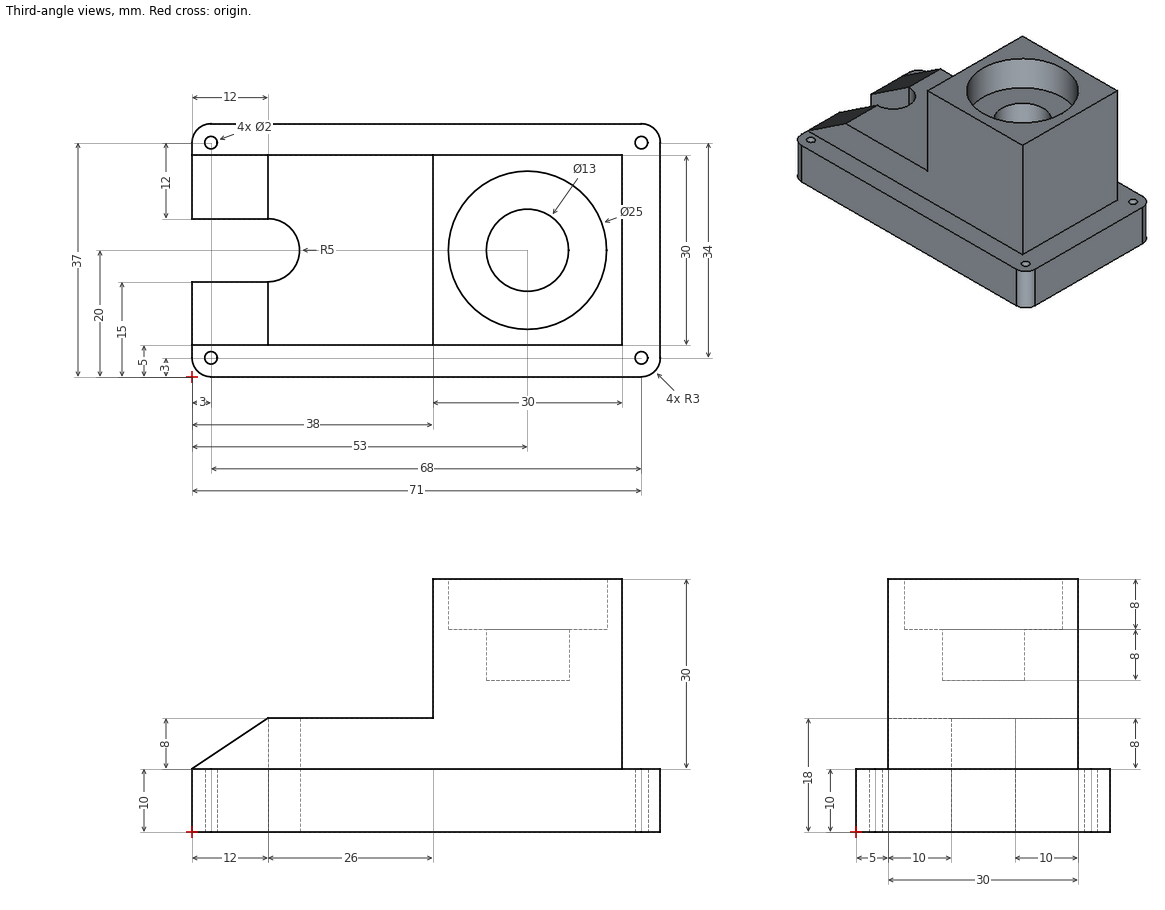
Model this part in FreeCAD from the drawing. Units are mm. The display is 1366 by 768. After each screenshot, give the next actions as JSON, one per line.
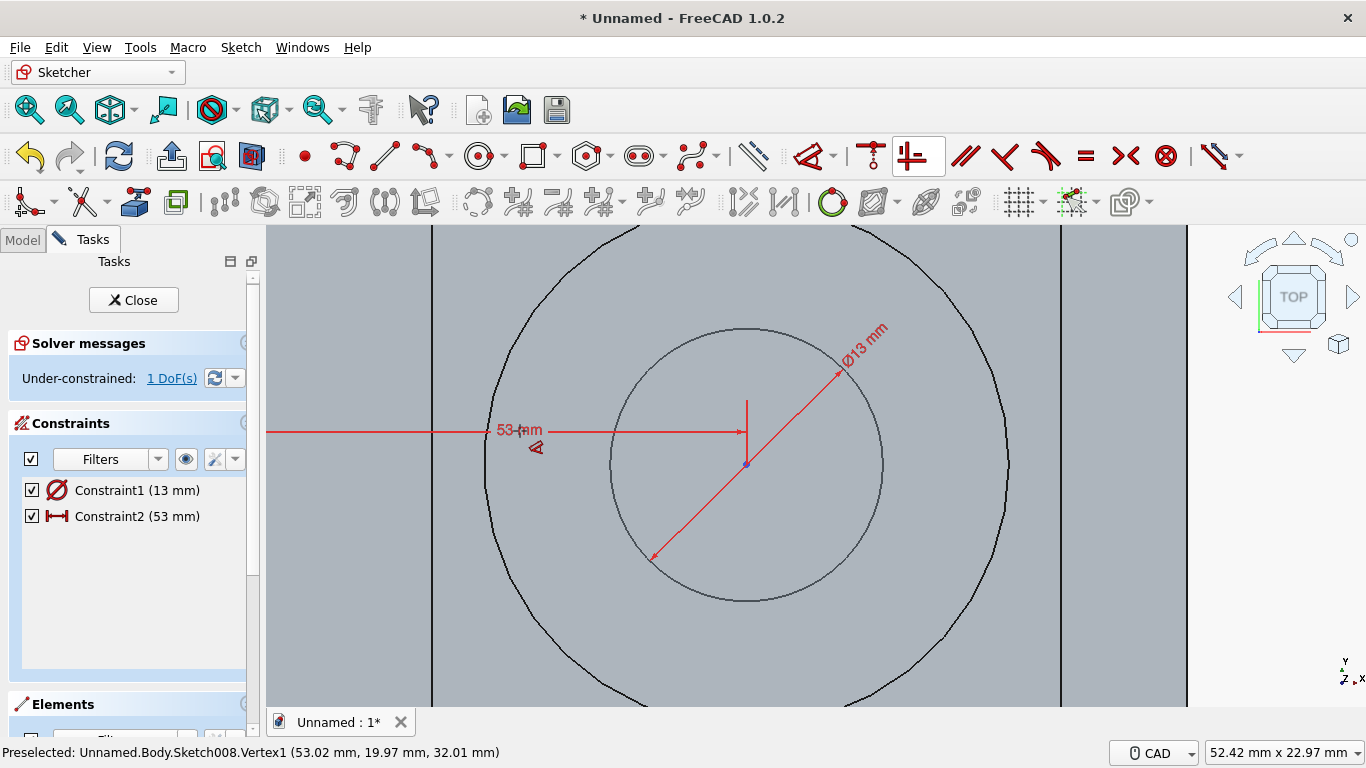
{"action": "left_click", "coordinate": [747, 465]}
{"action": "left_click", "coordinate": [781, 572]}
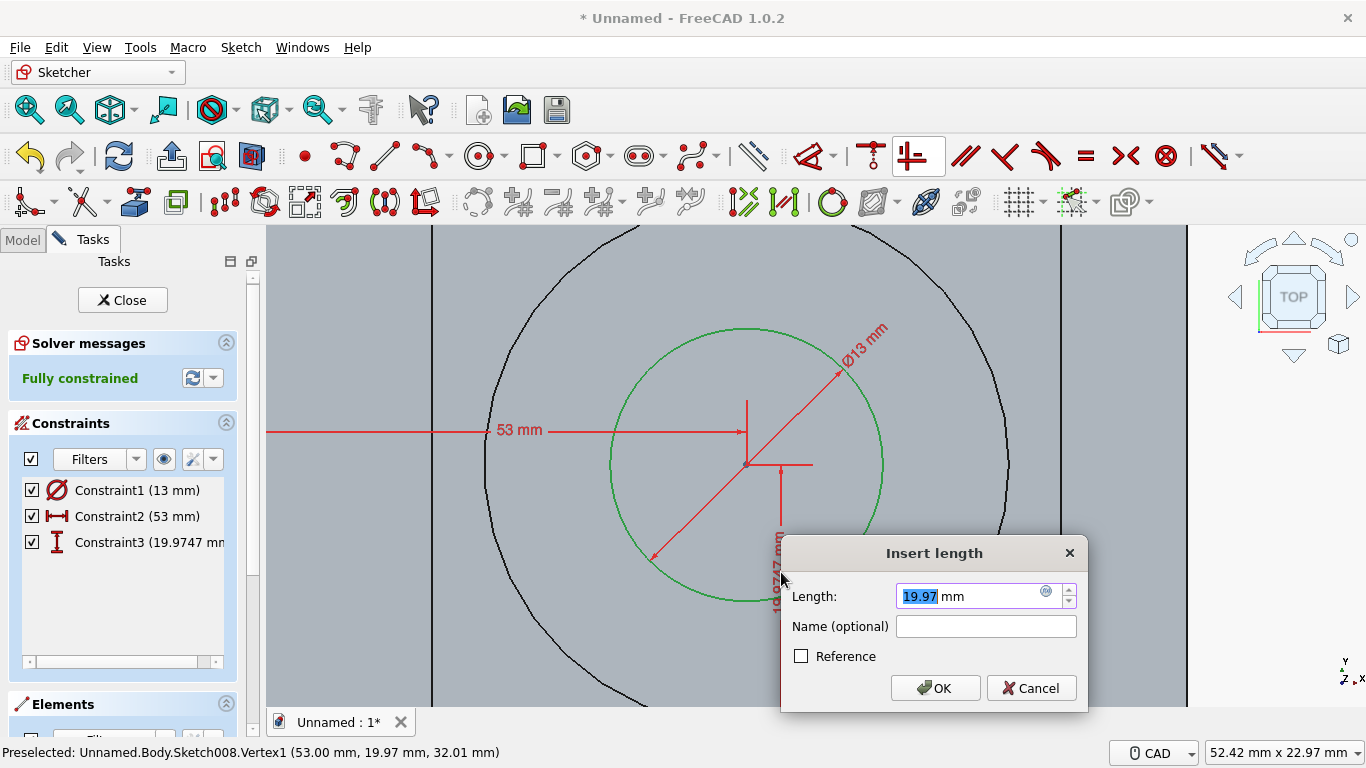
{"action": "type", "text": "20"}
{"action": "key", "text": "Return"}
{"action": "key", "text": "Escape"}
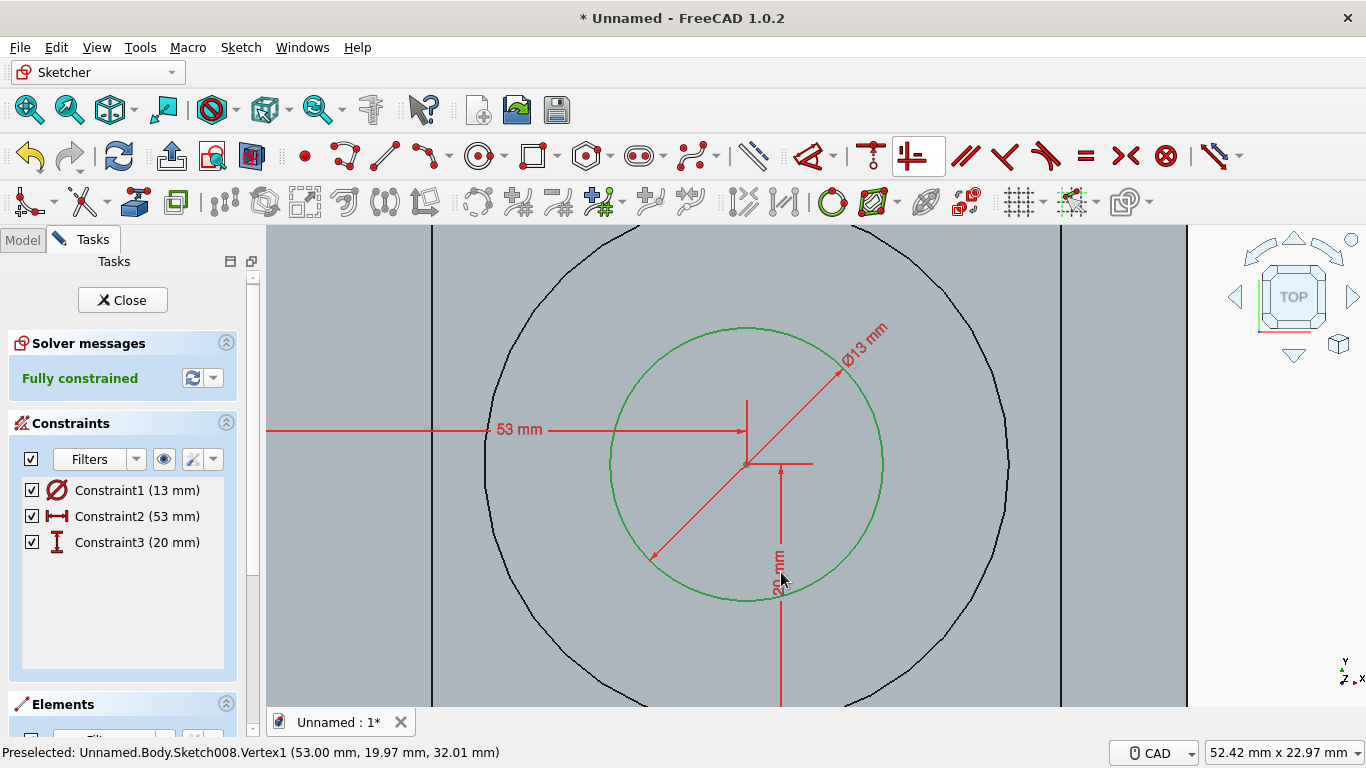
{"action": "left_click", "coordinate": [123, 300]}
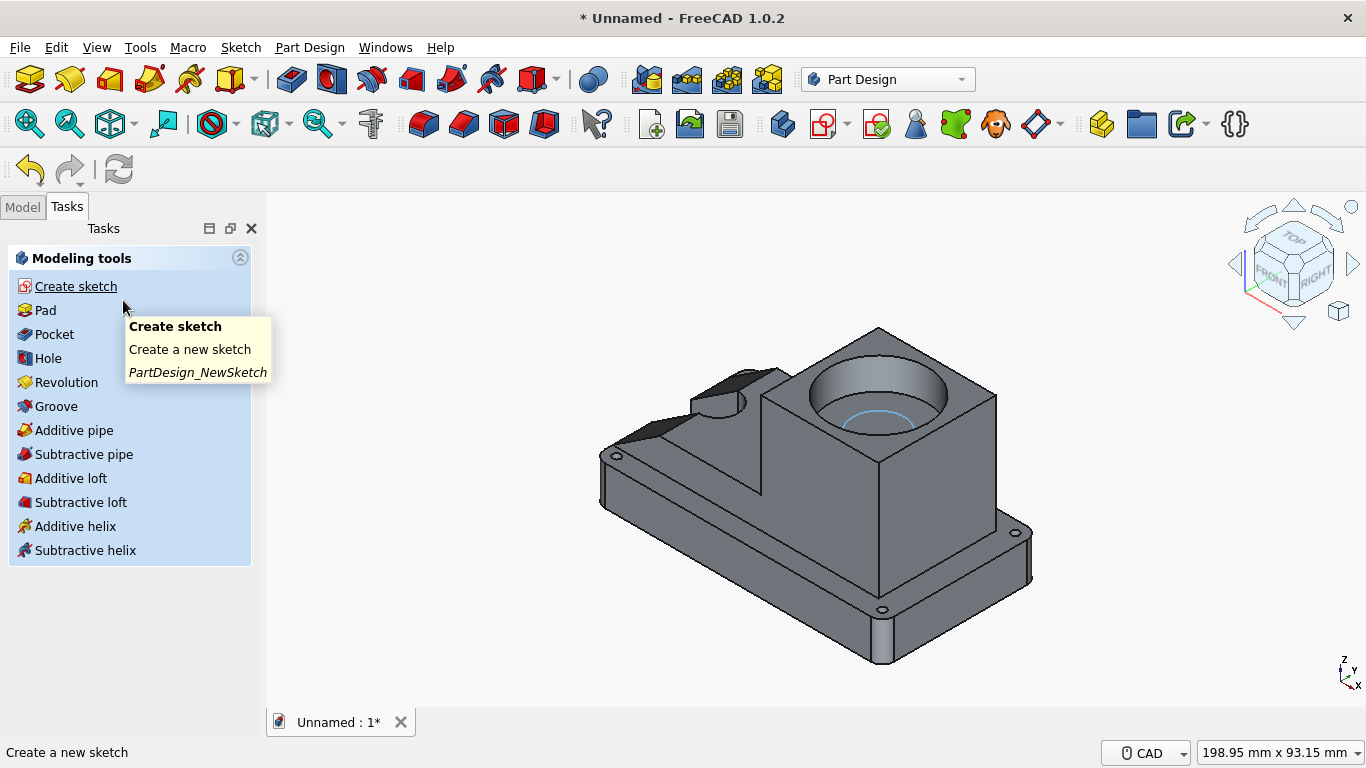
{"action": "left_click", "coordinate": [292, 80]}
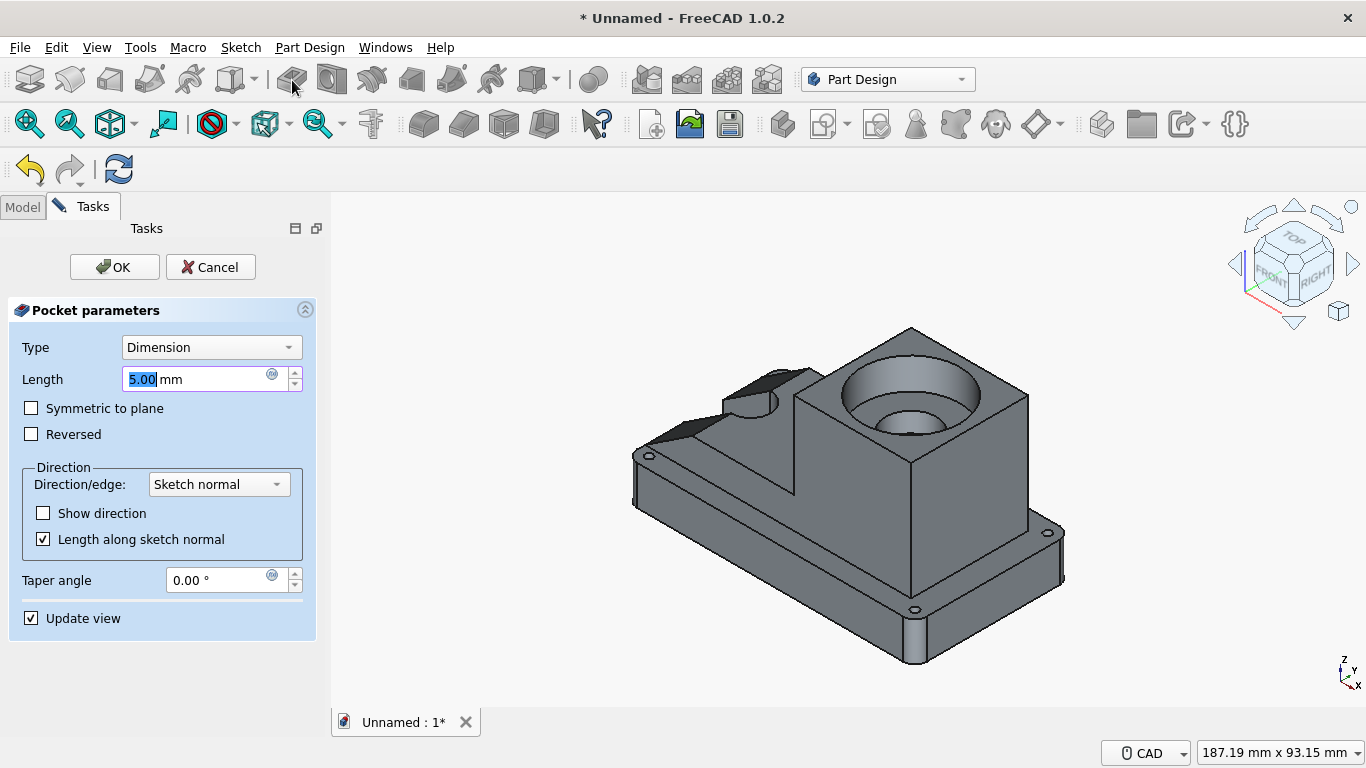
{"action": "type", "text": "8"}
{"action": "key", "text": "Tab"}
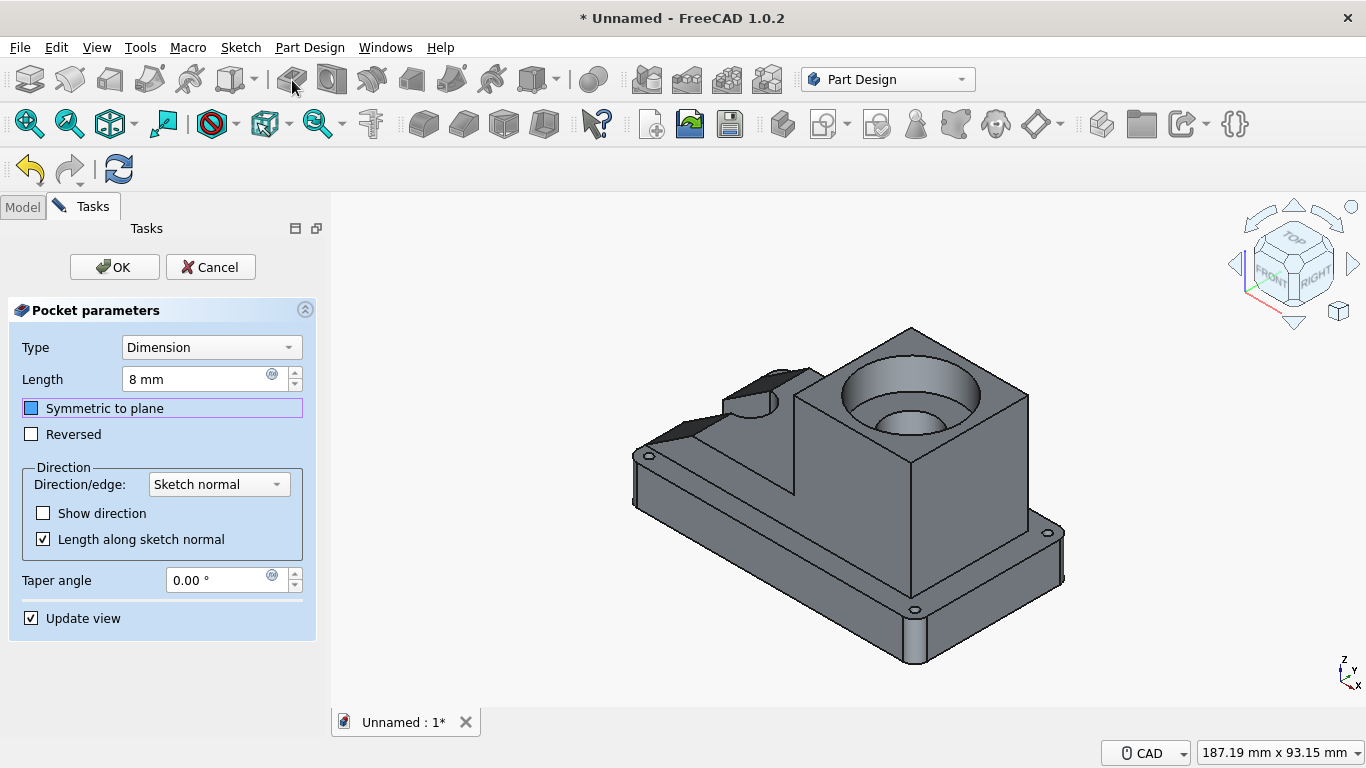
{"action": "left_click", "coordinate": [115, 267]}